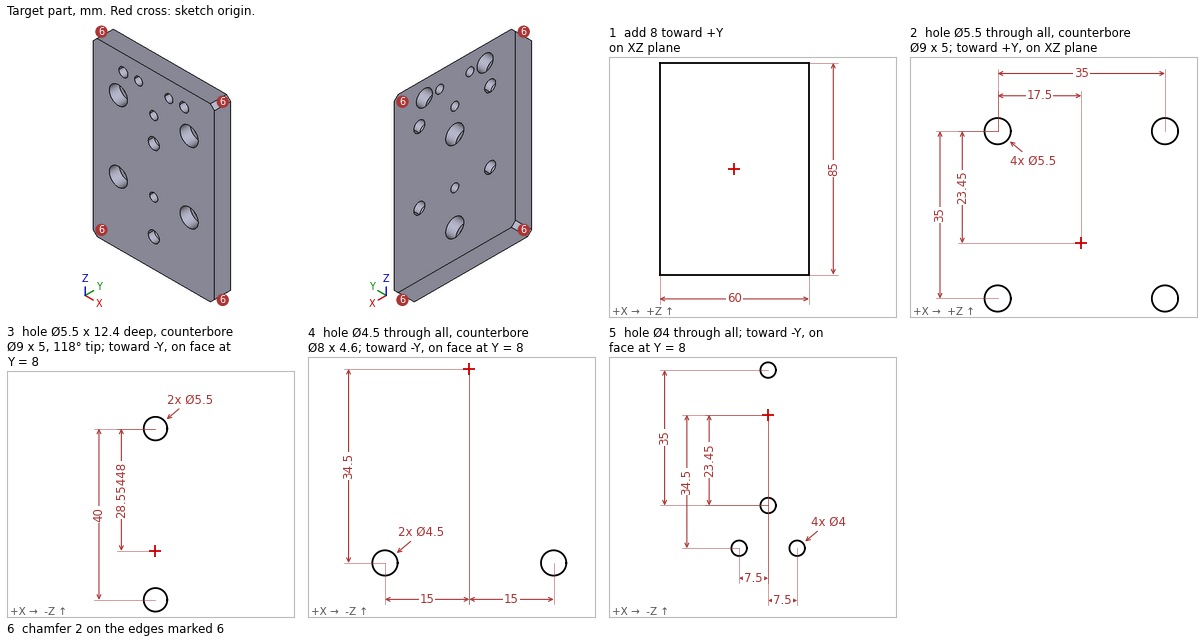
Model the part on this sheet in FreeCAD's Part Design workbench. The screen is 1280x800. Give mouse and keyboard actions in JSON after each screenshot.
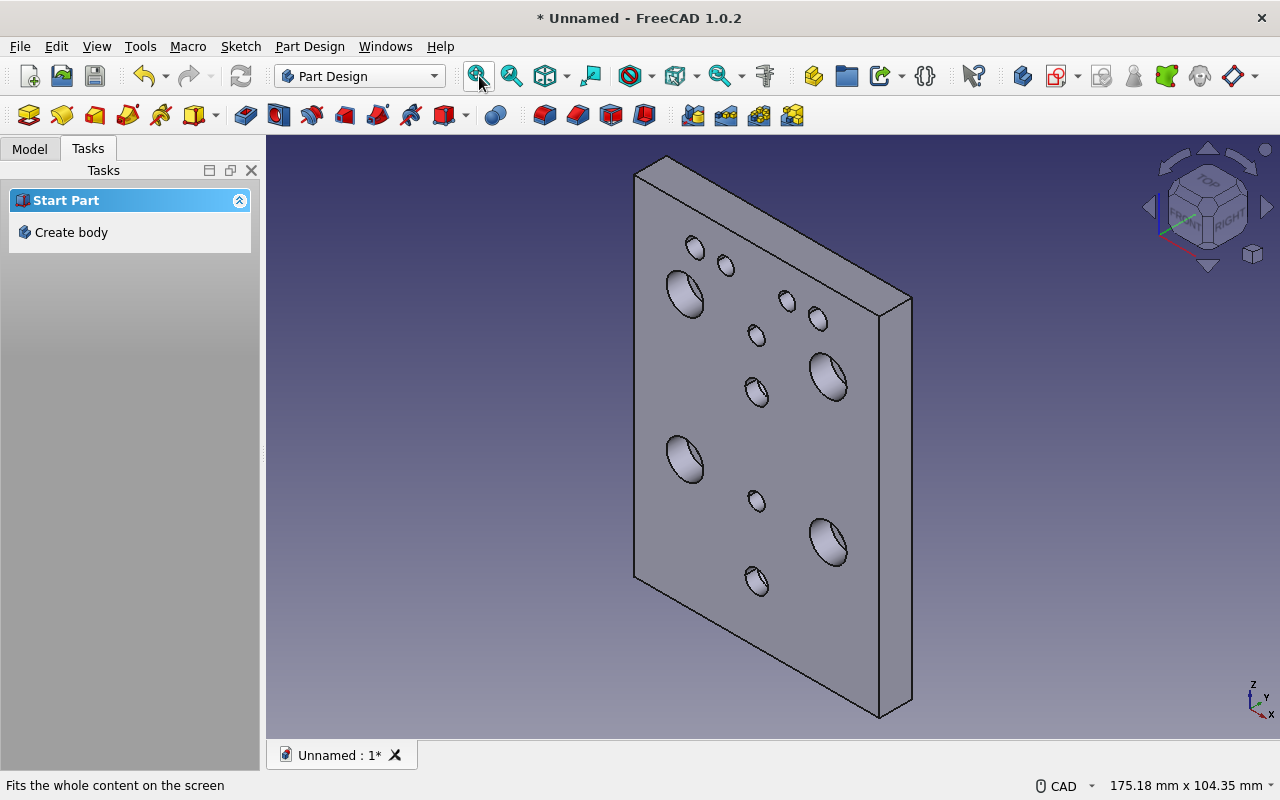
{"action": "left_click", "coordinate": [896, 306]}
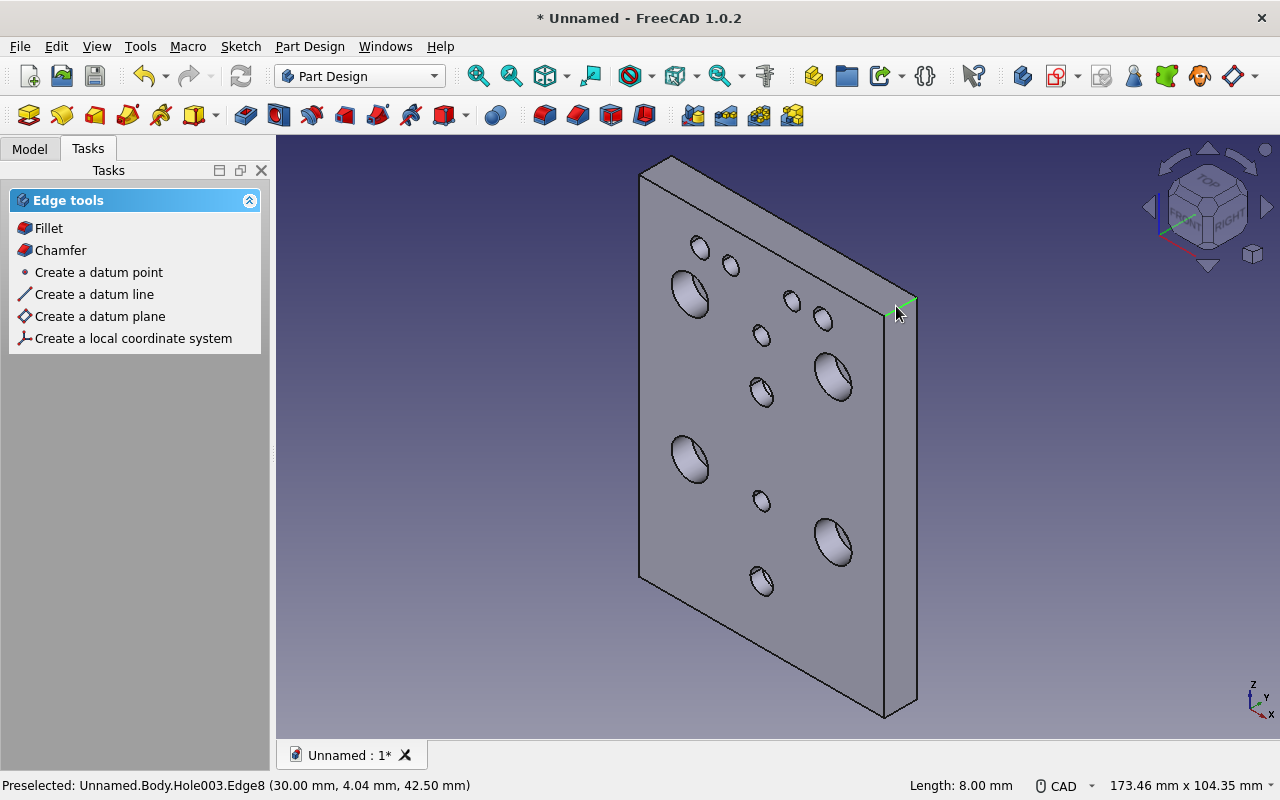
{"action": "key", "text": "2"}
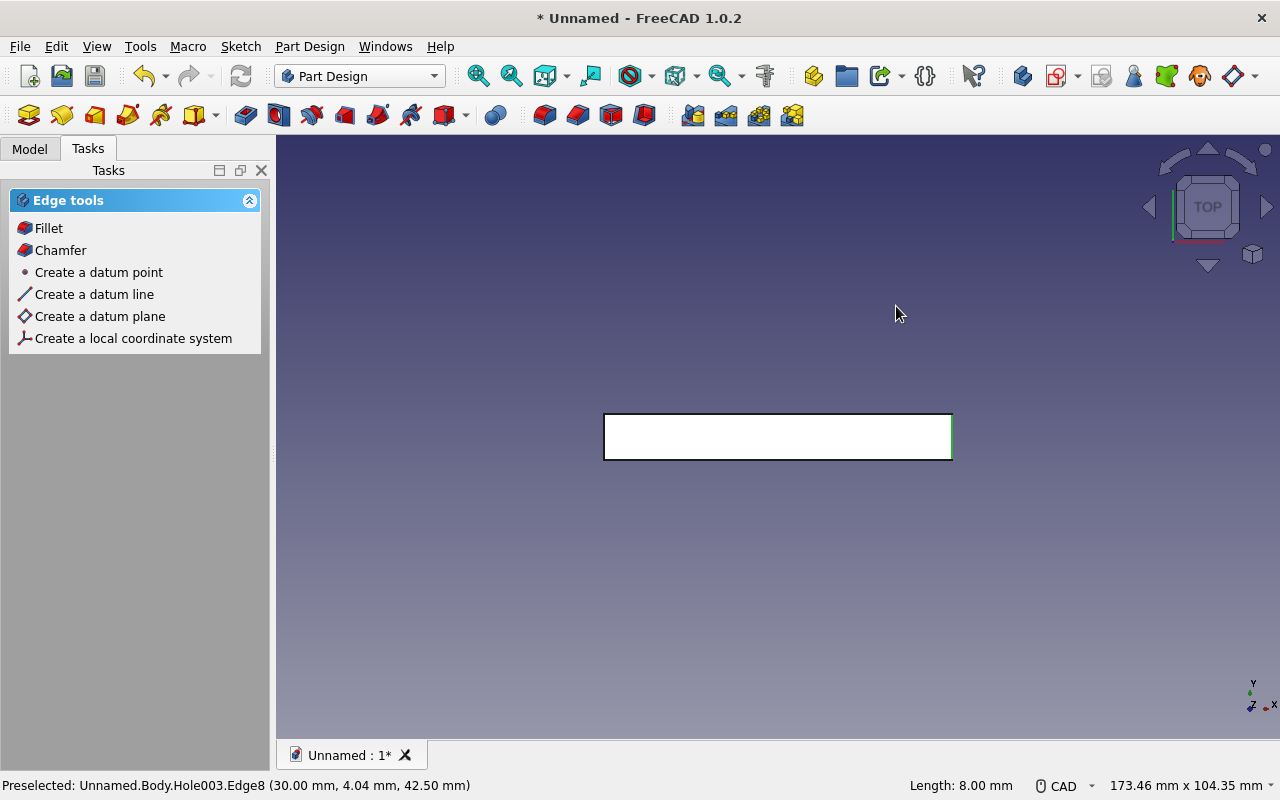
{"action": "left_click", "coordinate": [479, 76]}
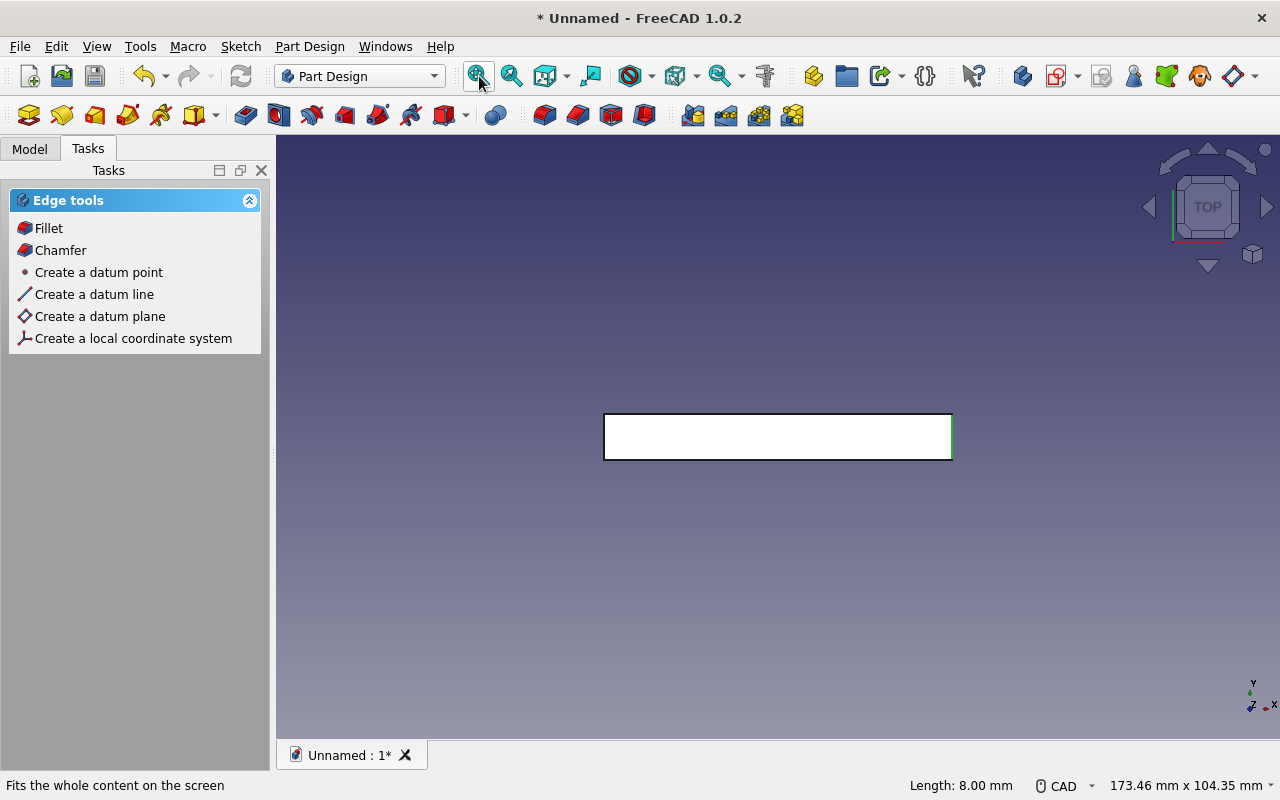
{"action": "left_click", "coordinate": [604, 436], "text": "ctrl"}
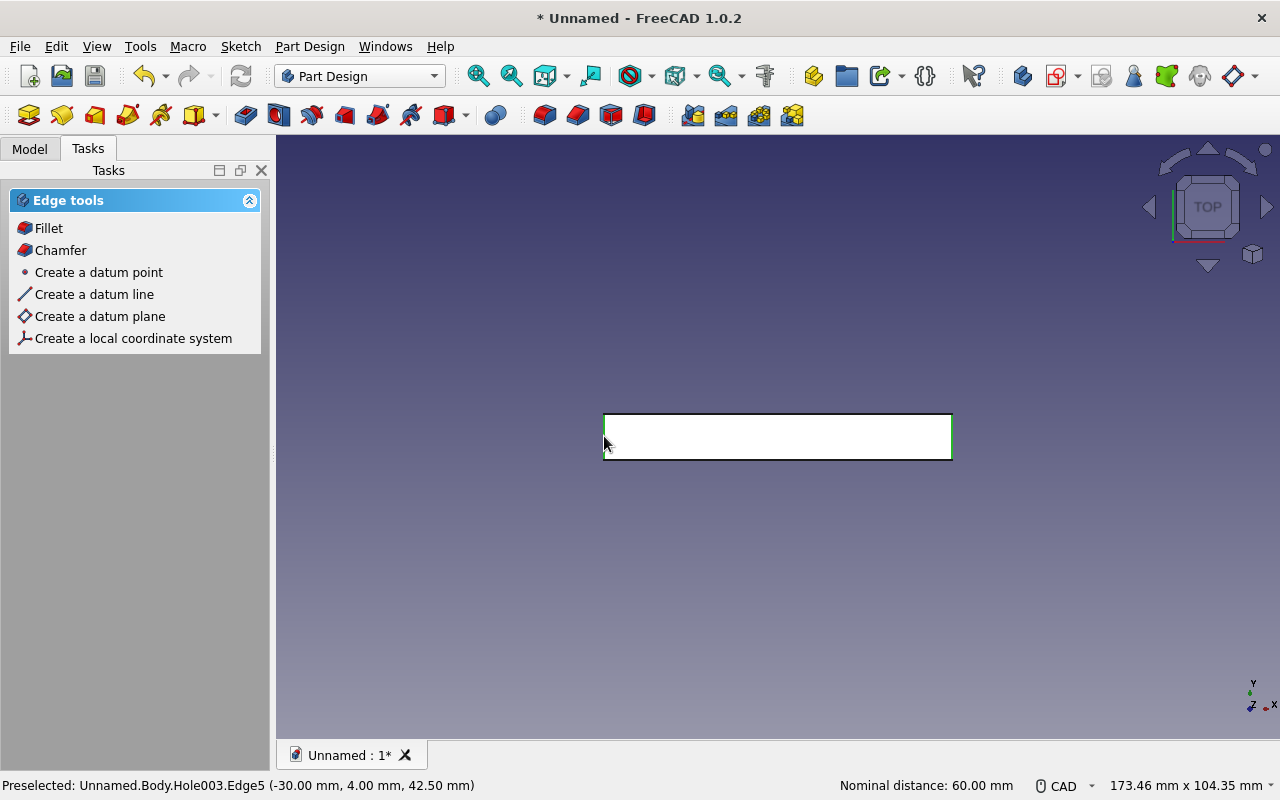
{"action": "key", "text": "1"}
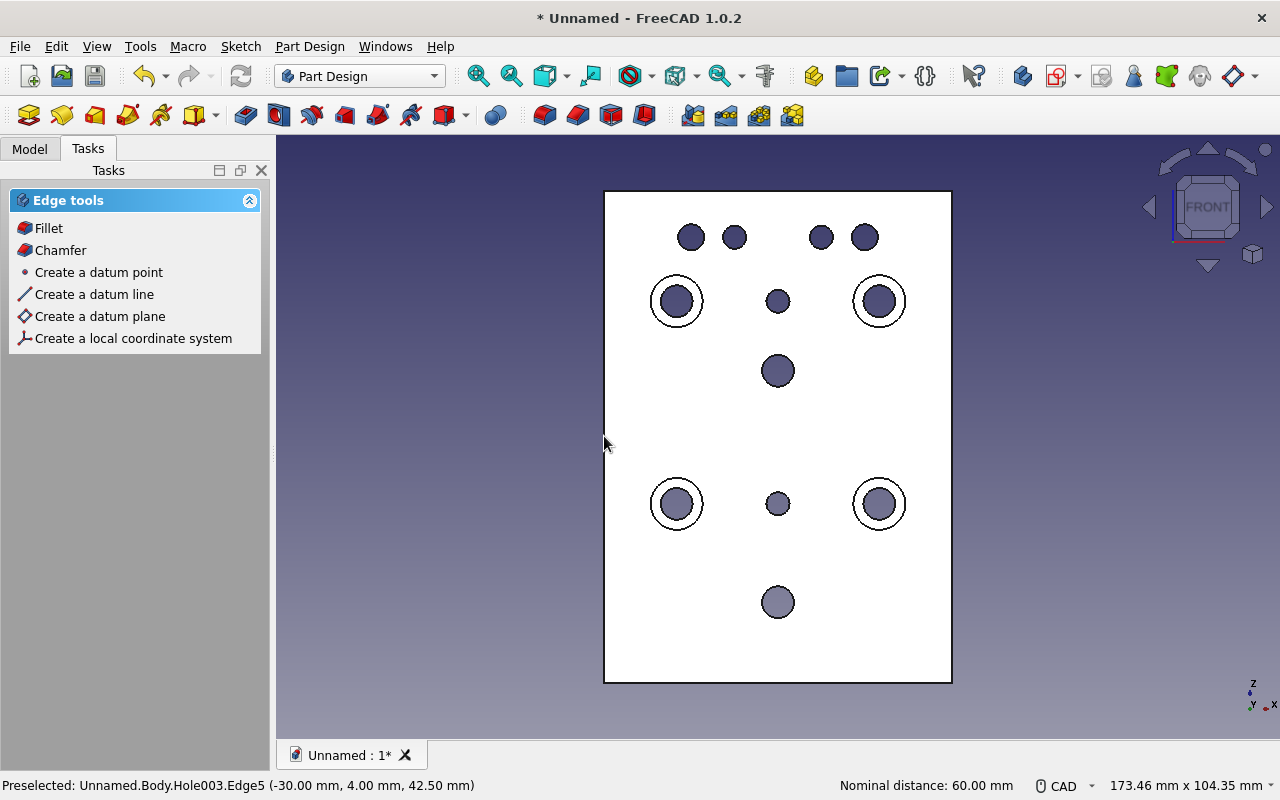
{"action": "key", "text": "3"}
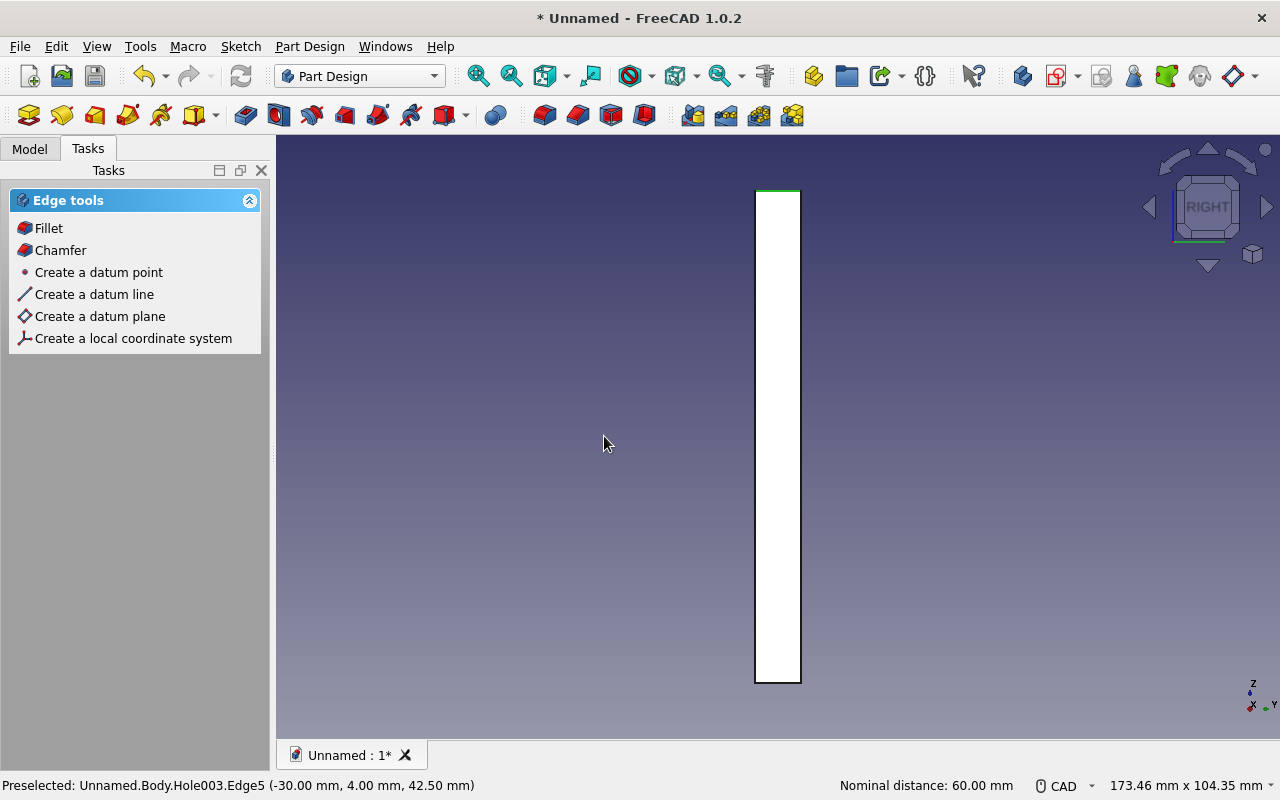
{"action": "left_click", "coordinate": [778, 682], "text": "ctrl"}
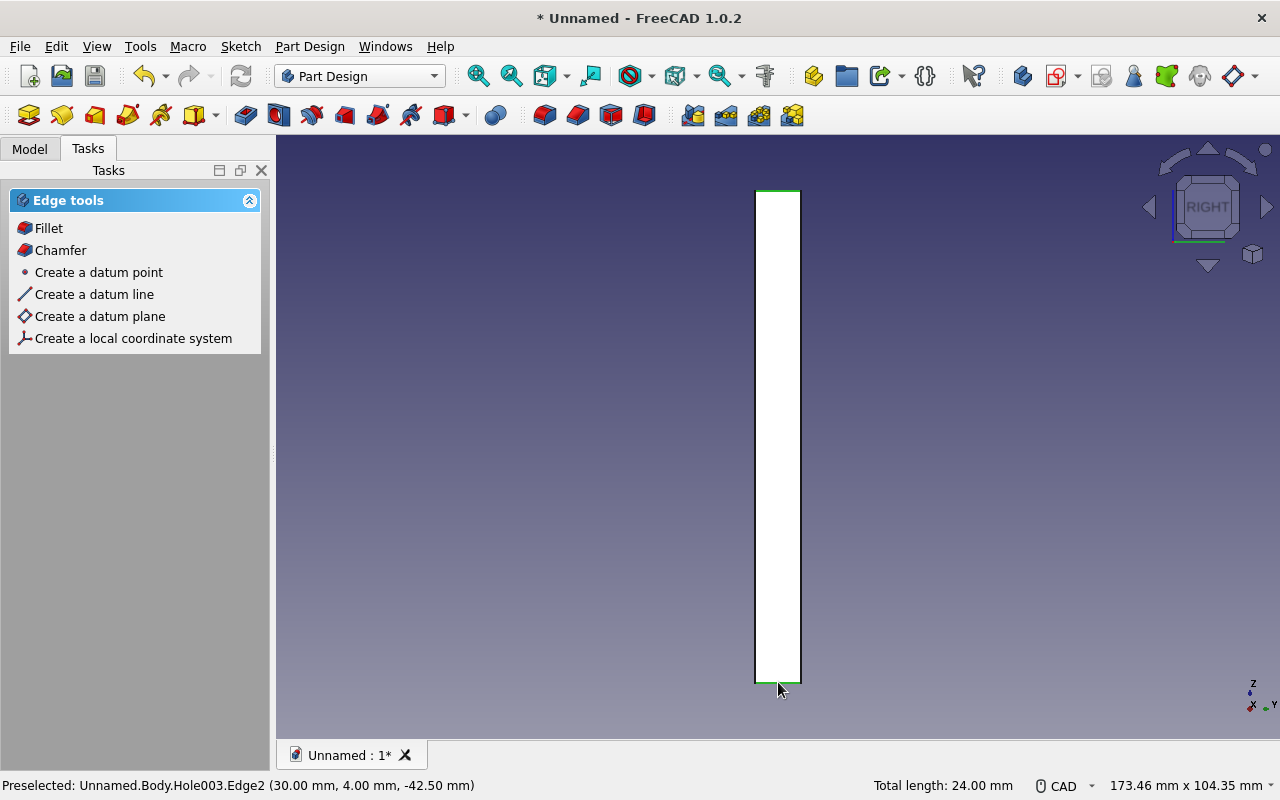
{"action": "key", "text": "5"}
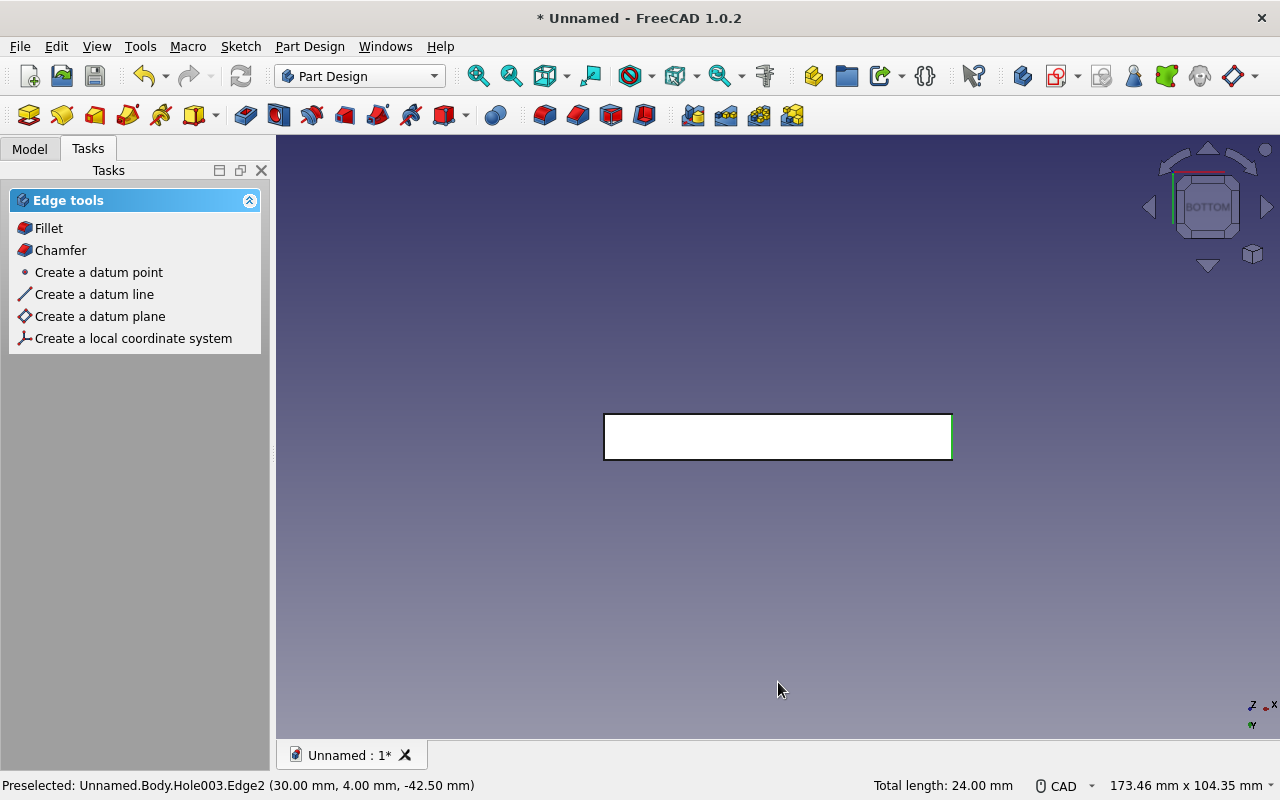
{"action": "left_click", "coordinate": [479, 76]}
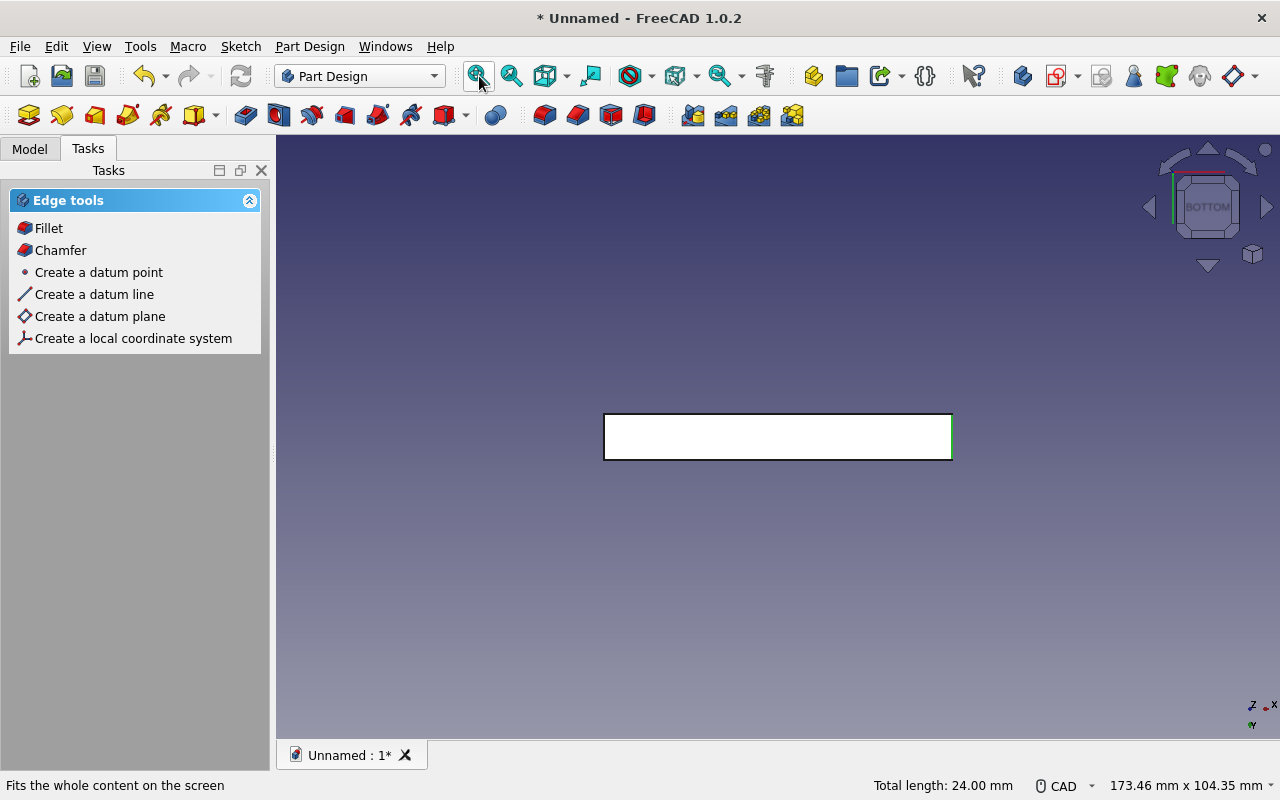
{"action": "left_click", "coordinate": [604, 436], "text": "ctrl"}